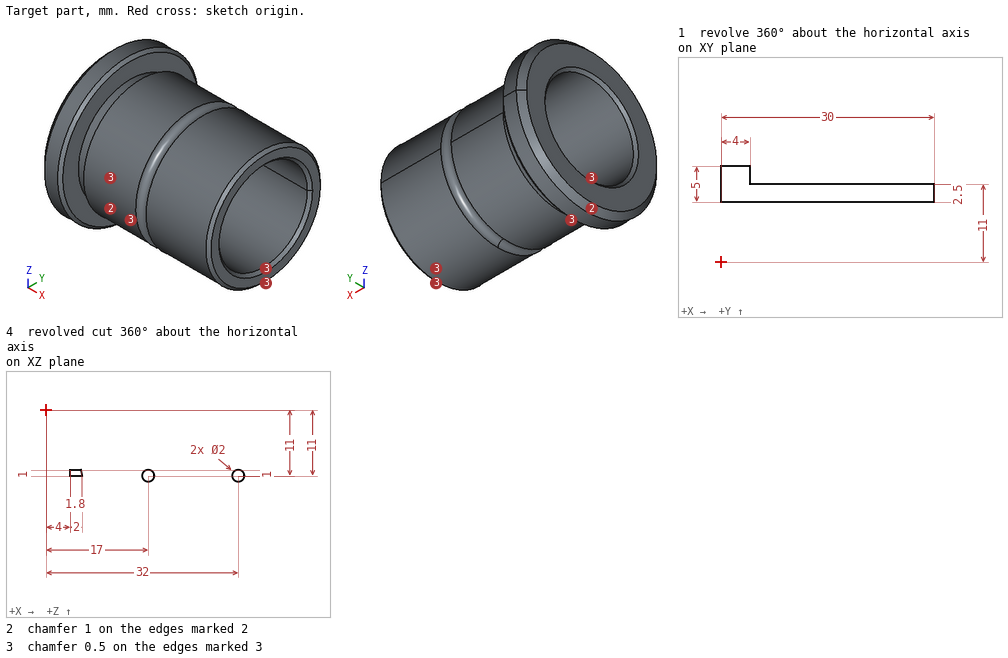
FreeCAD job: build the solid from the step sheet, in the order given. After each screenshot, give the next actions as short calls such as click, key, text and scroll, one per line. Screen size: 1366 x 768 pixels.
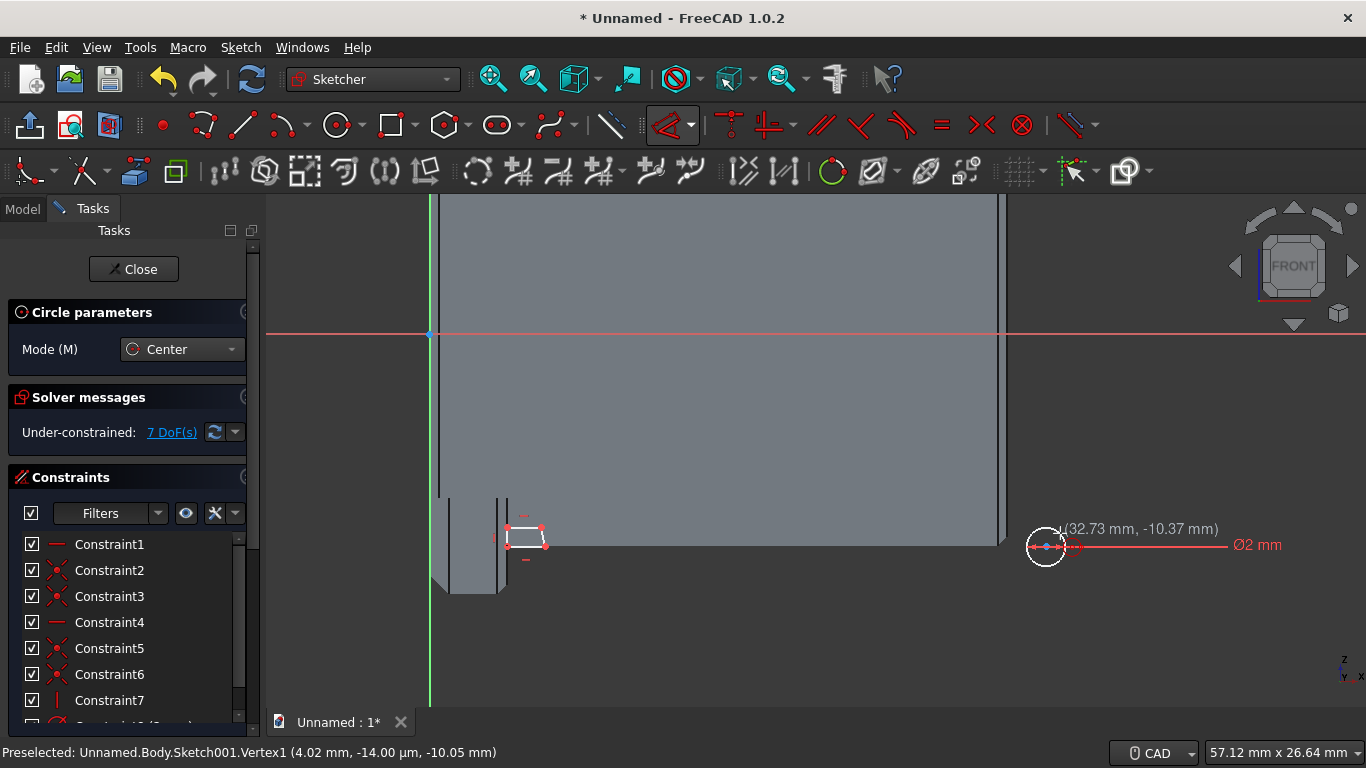
click(757, 546)
move(771, 533)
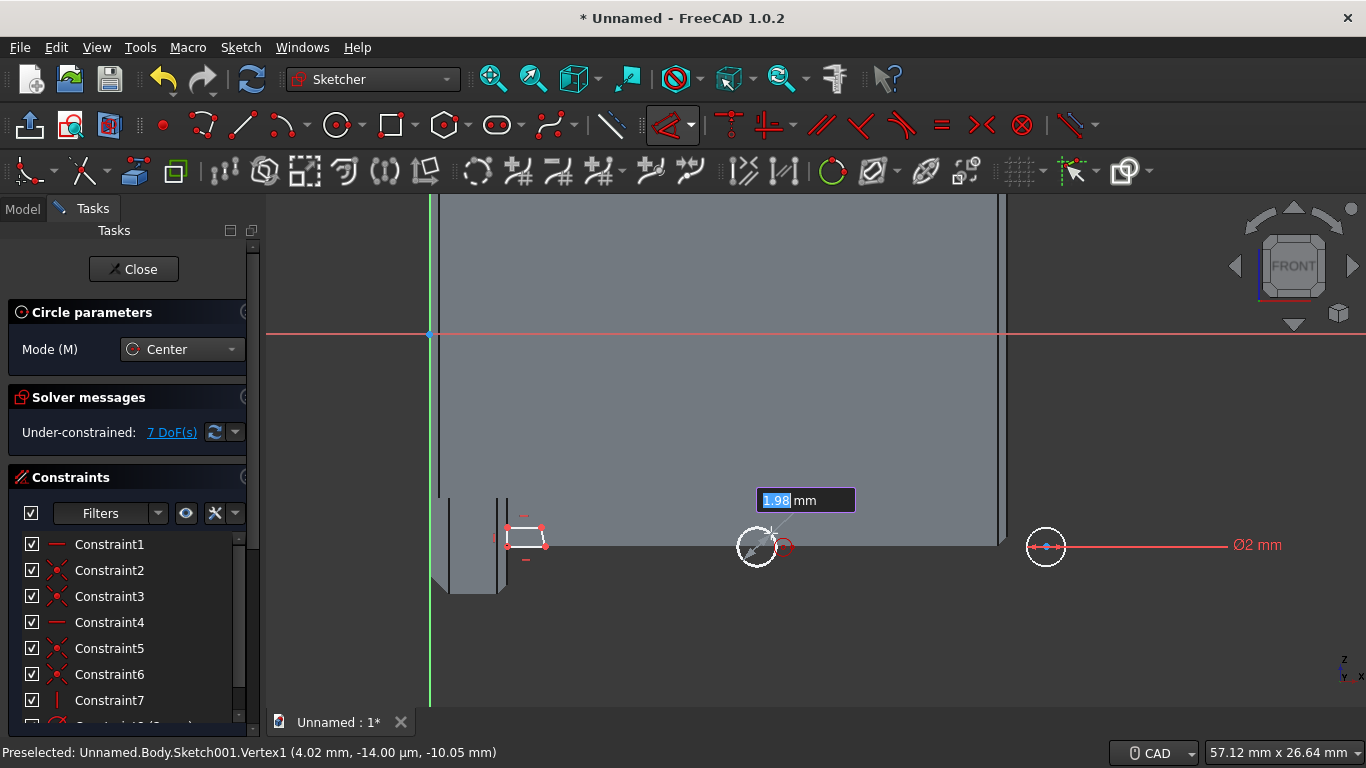
text(2)
key(Return)
key(Escape)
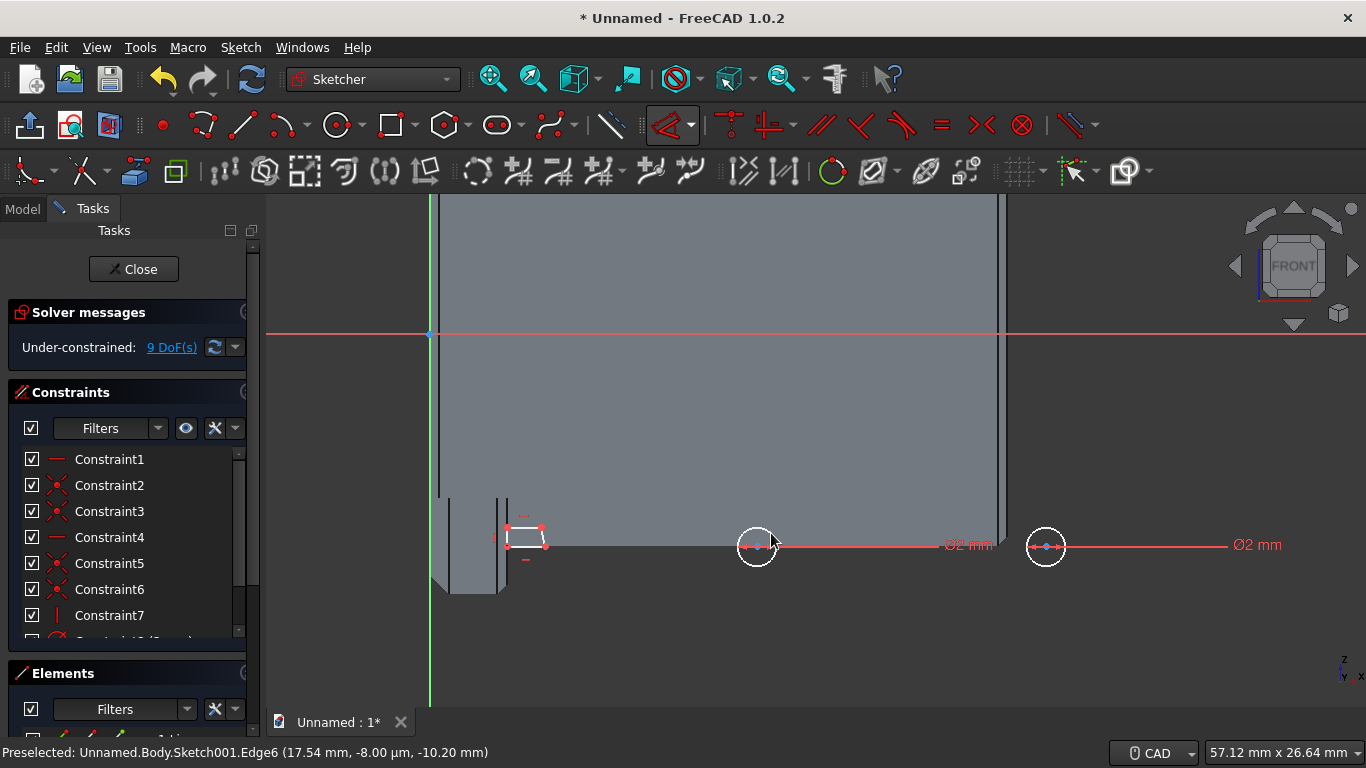
scroll(534, 547, up, 2)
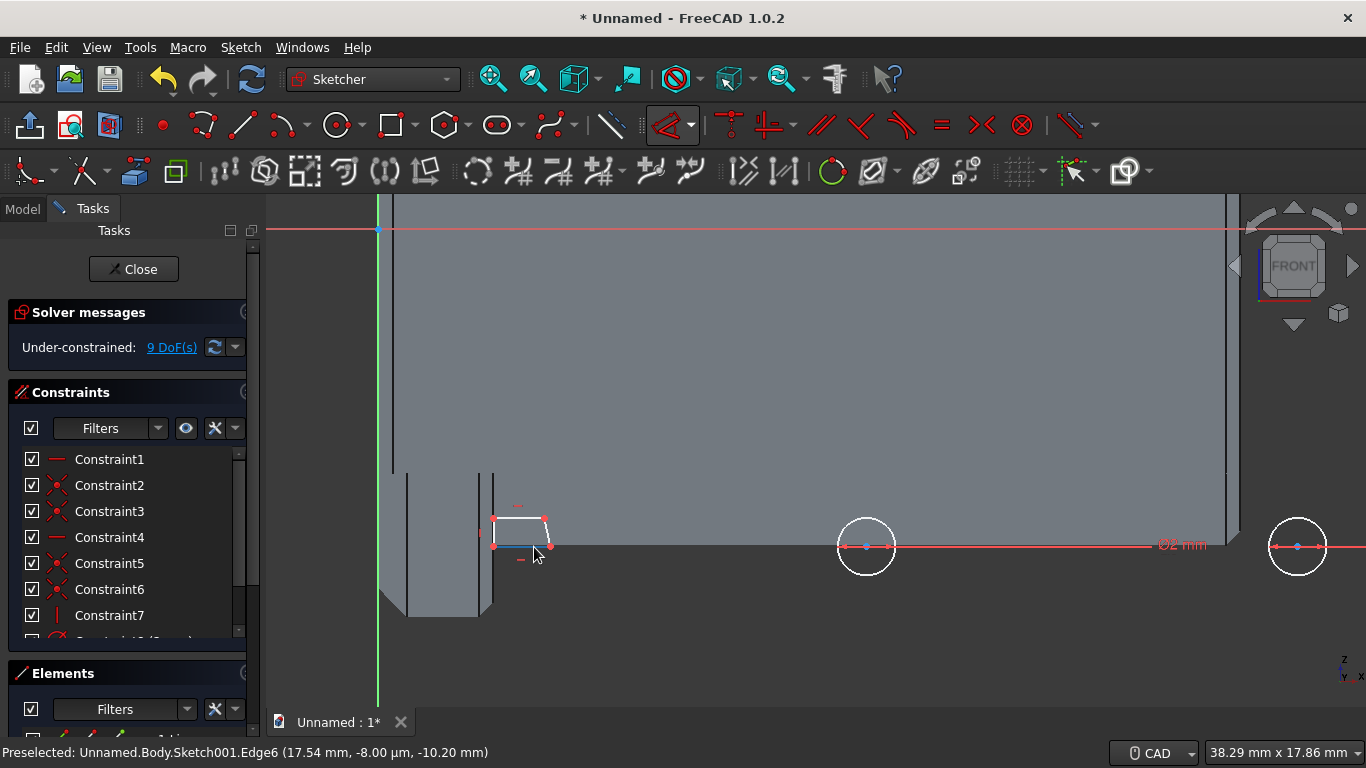
click(533, 547)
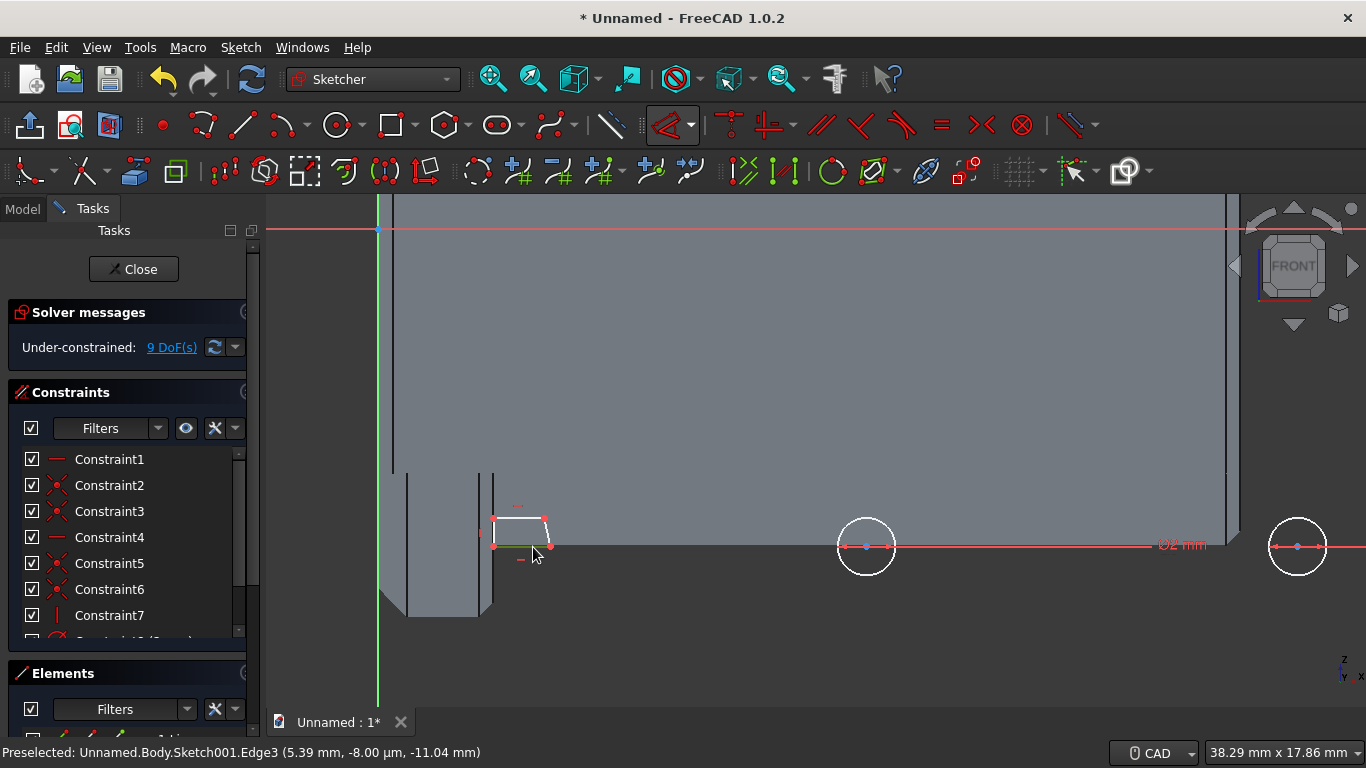
key(l)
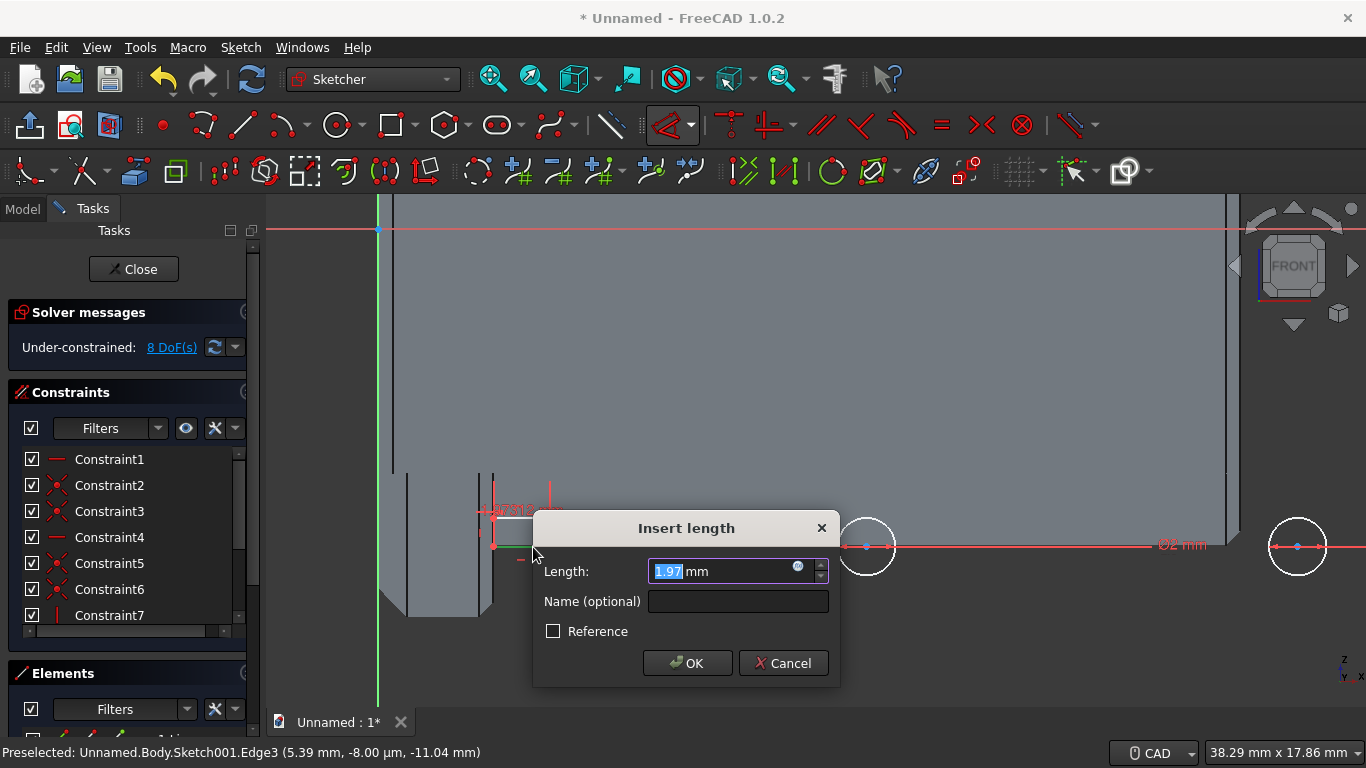
text(2)
key(Return)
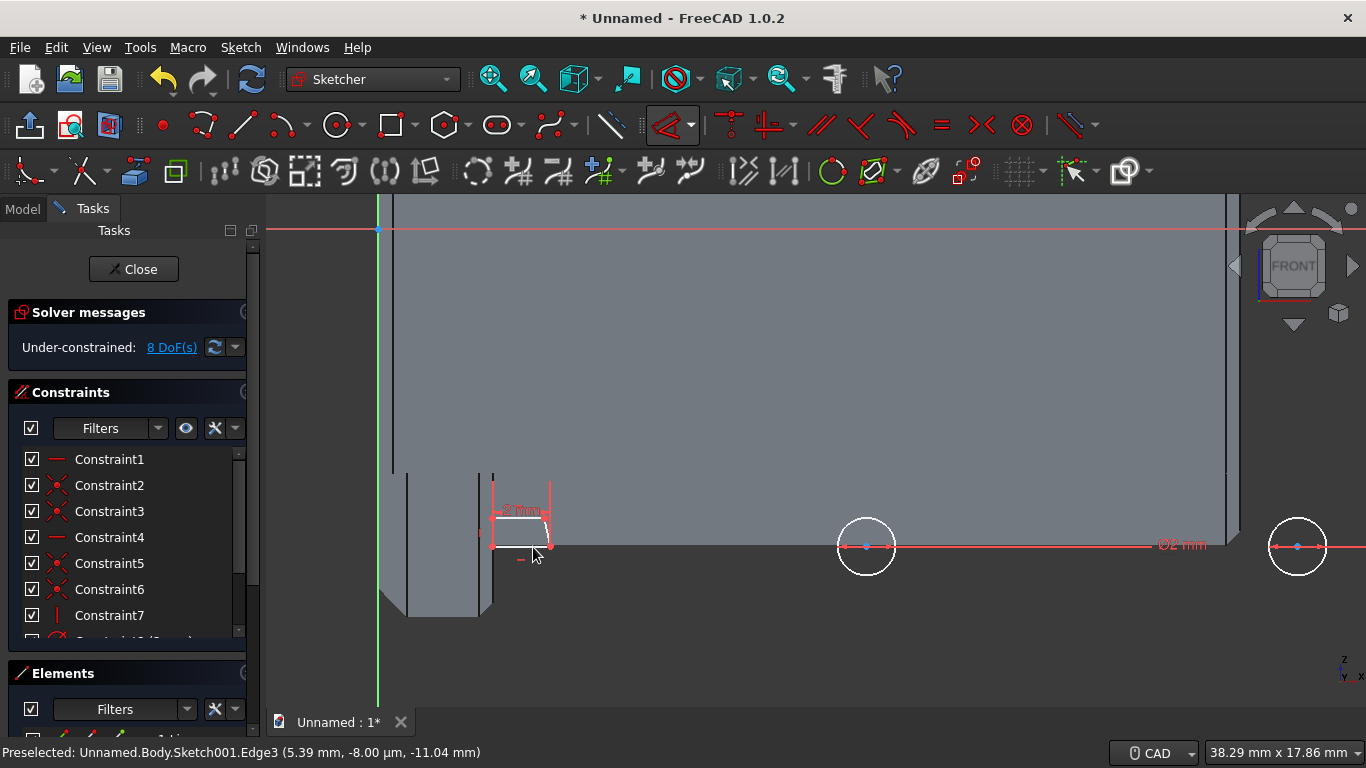
scroll(493, 535, up, 2)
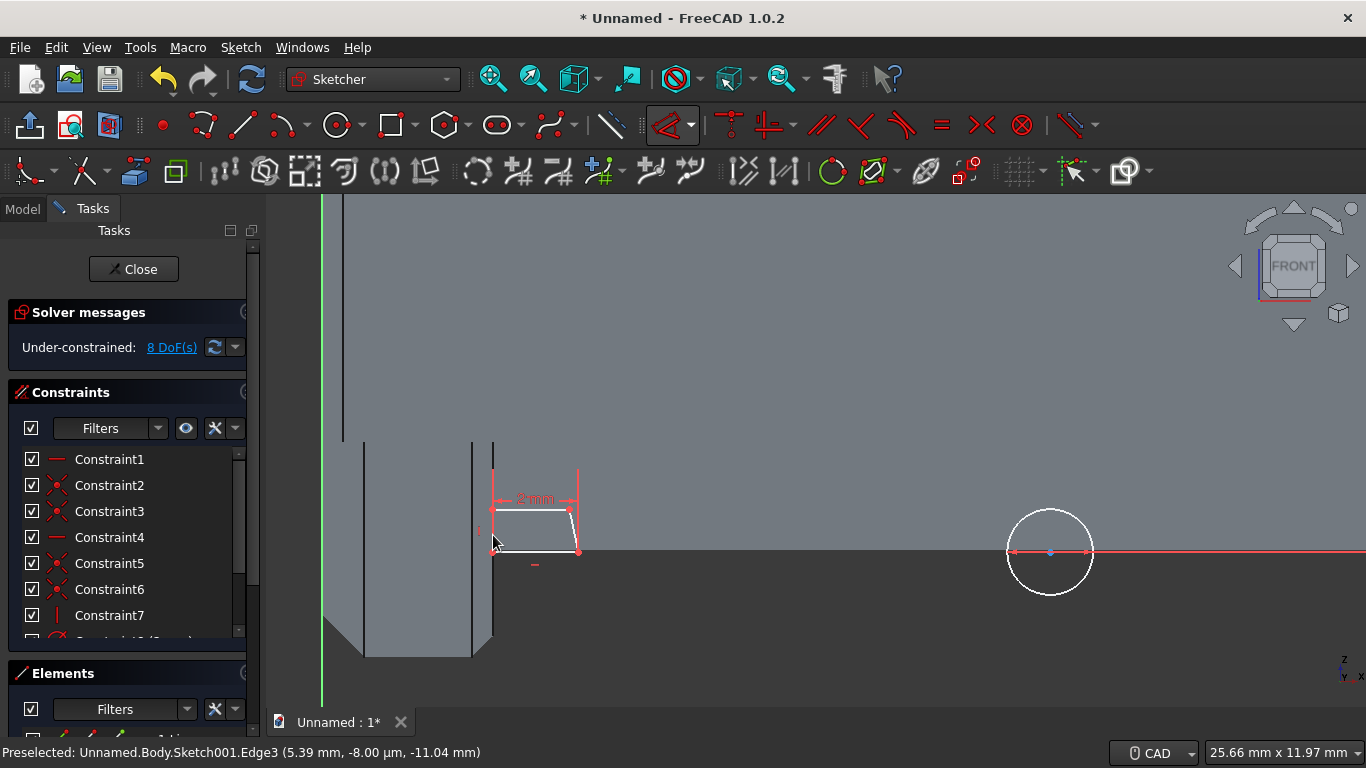
click(493, 535)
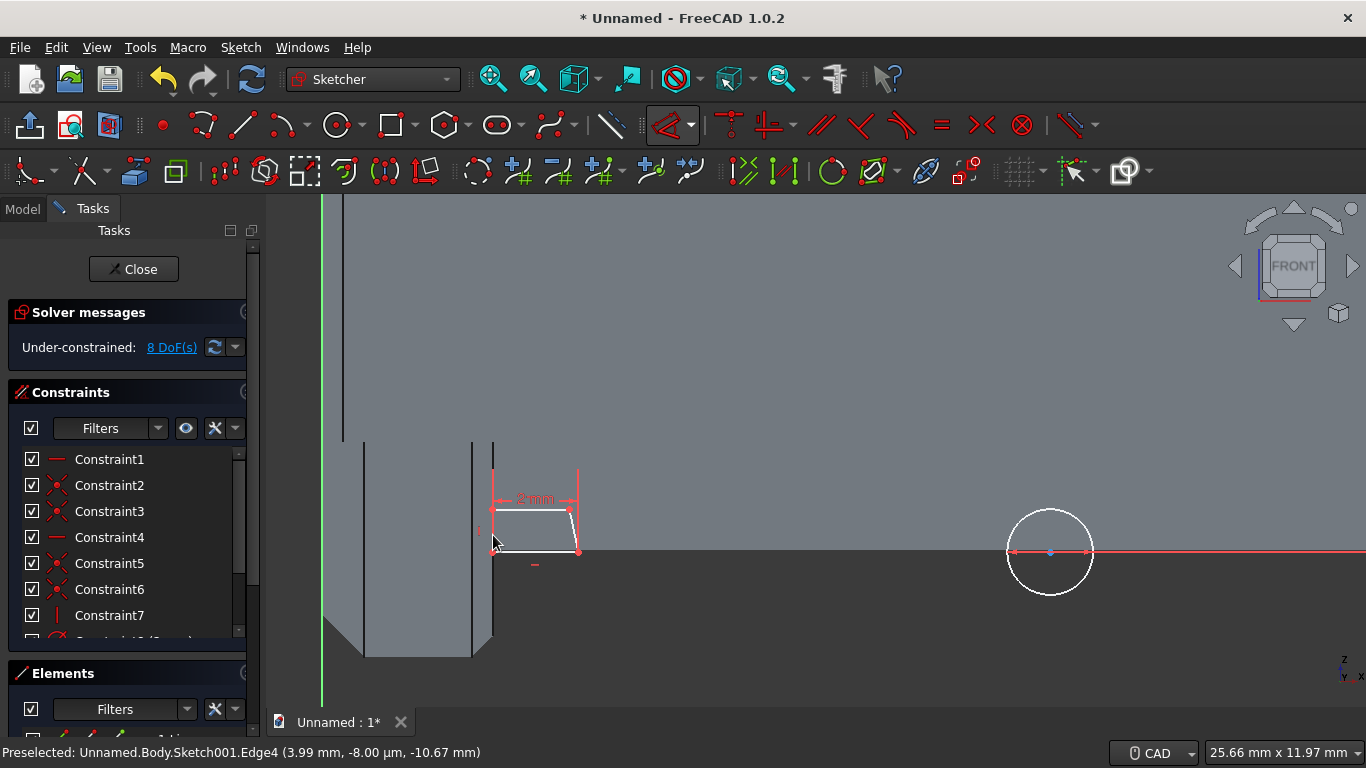
key(i)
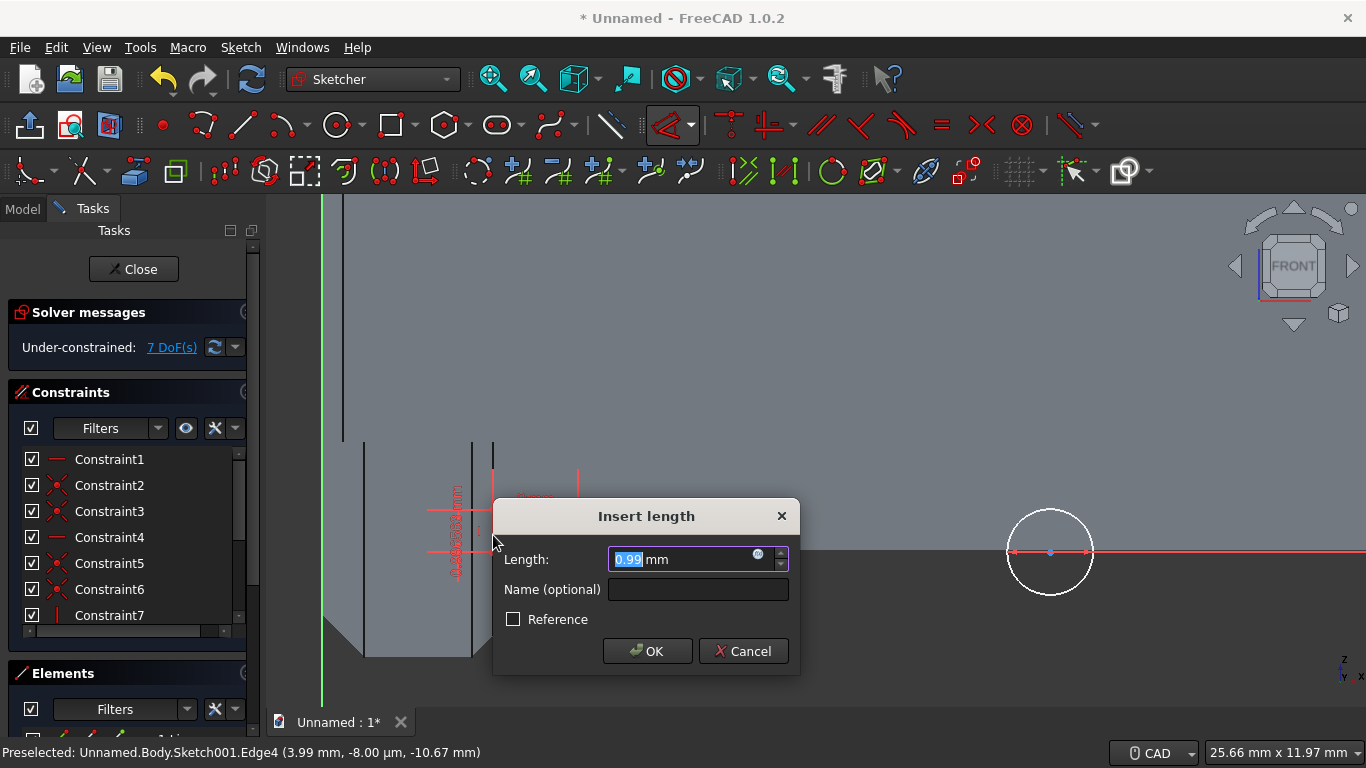
text(1)
key(Return)